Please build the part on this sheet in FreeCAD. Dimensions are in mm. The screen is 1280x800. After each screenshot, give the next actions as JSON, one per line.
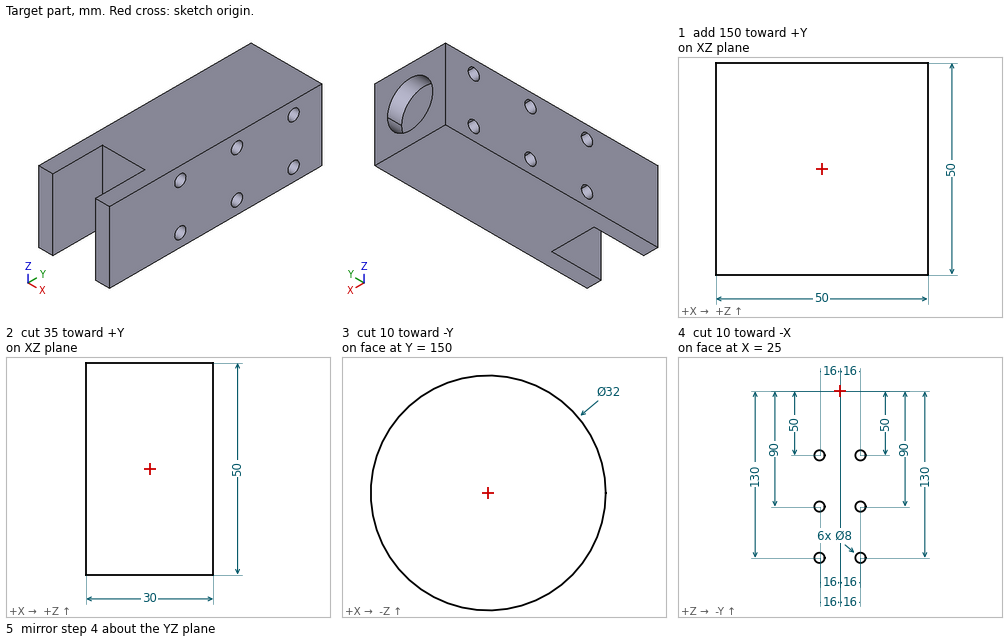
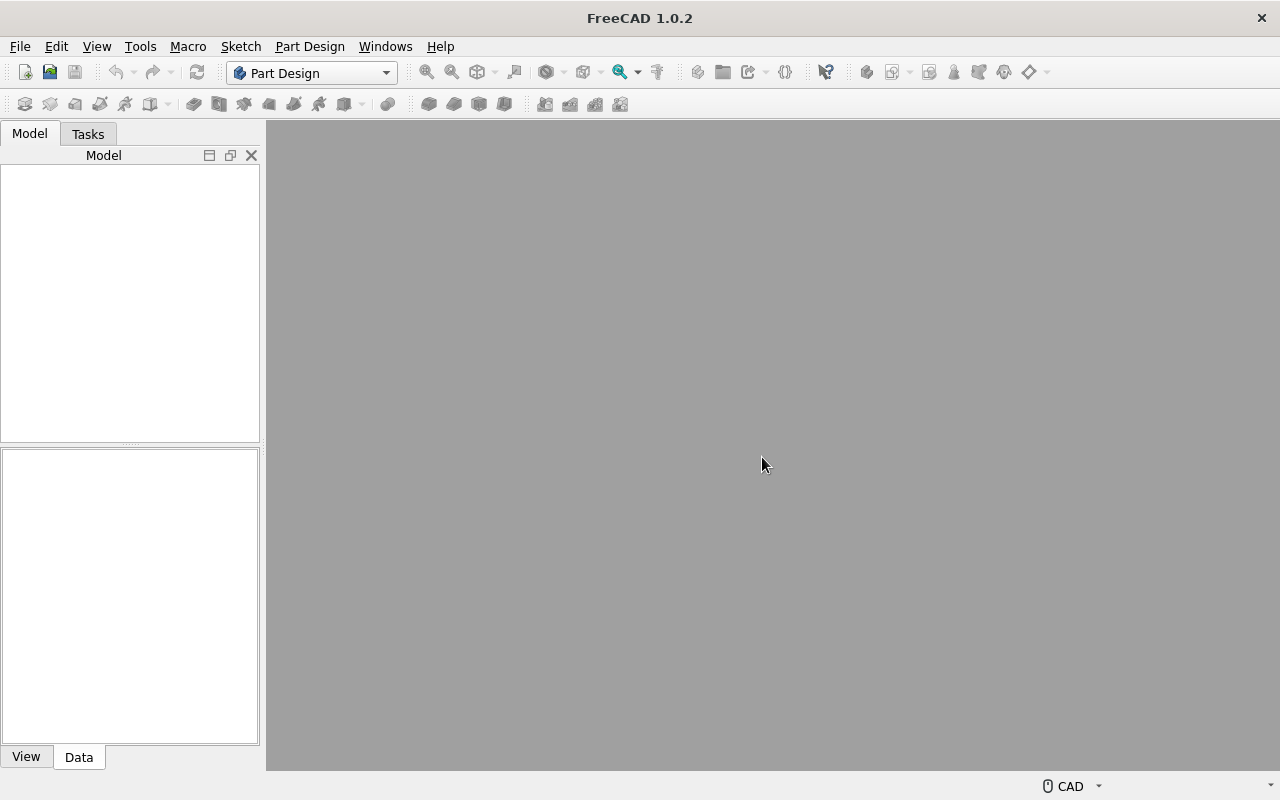
{"action": "left_click", "coordinate": [25, 72]}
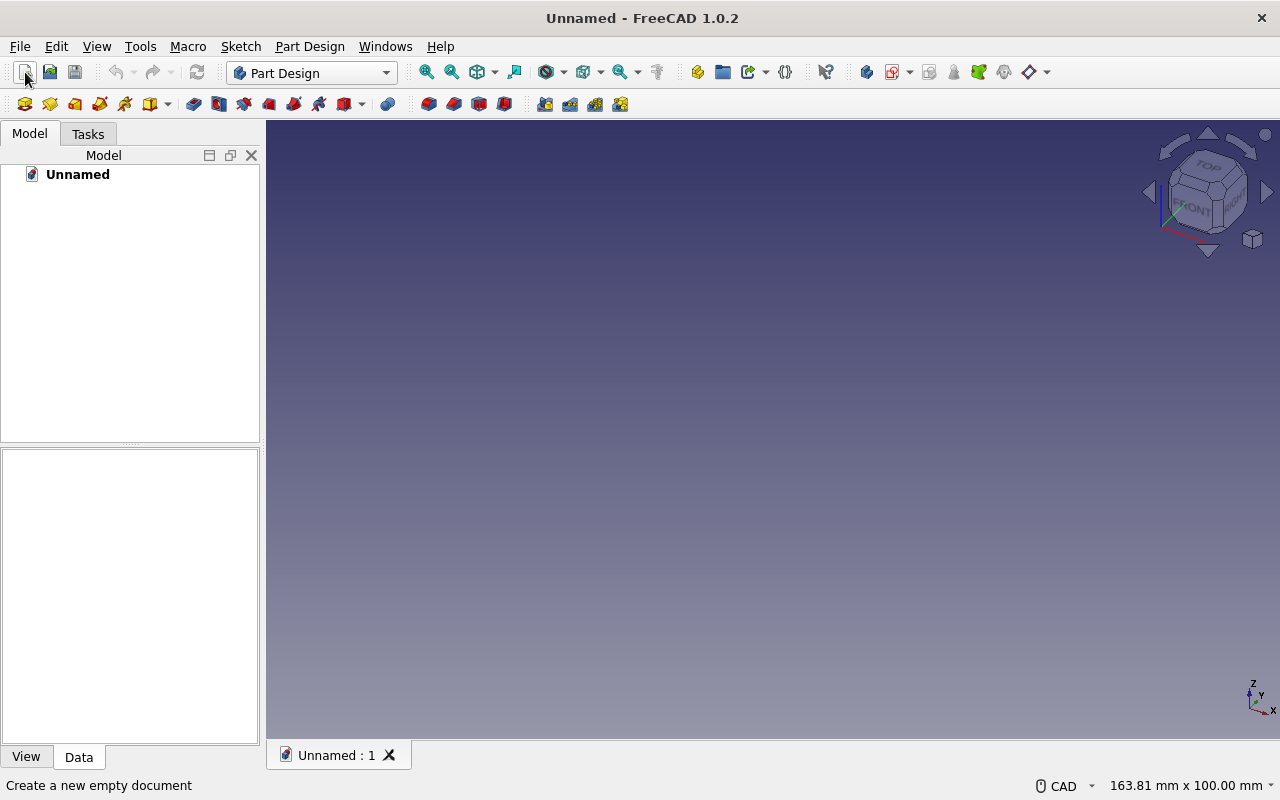
{"action": "left_click", "coordinate": [892, 72]}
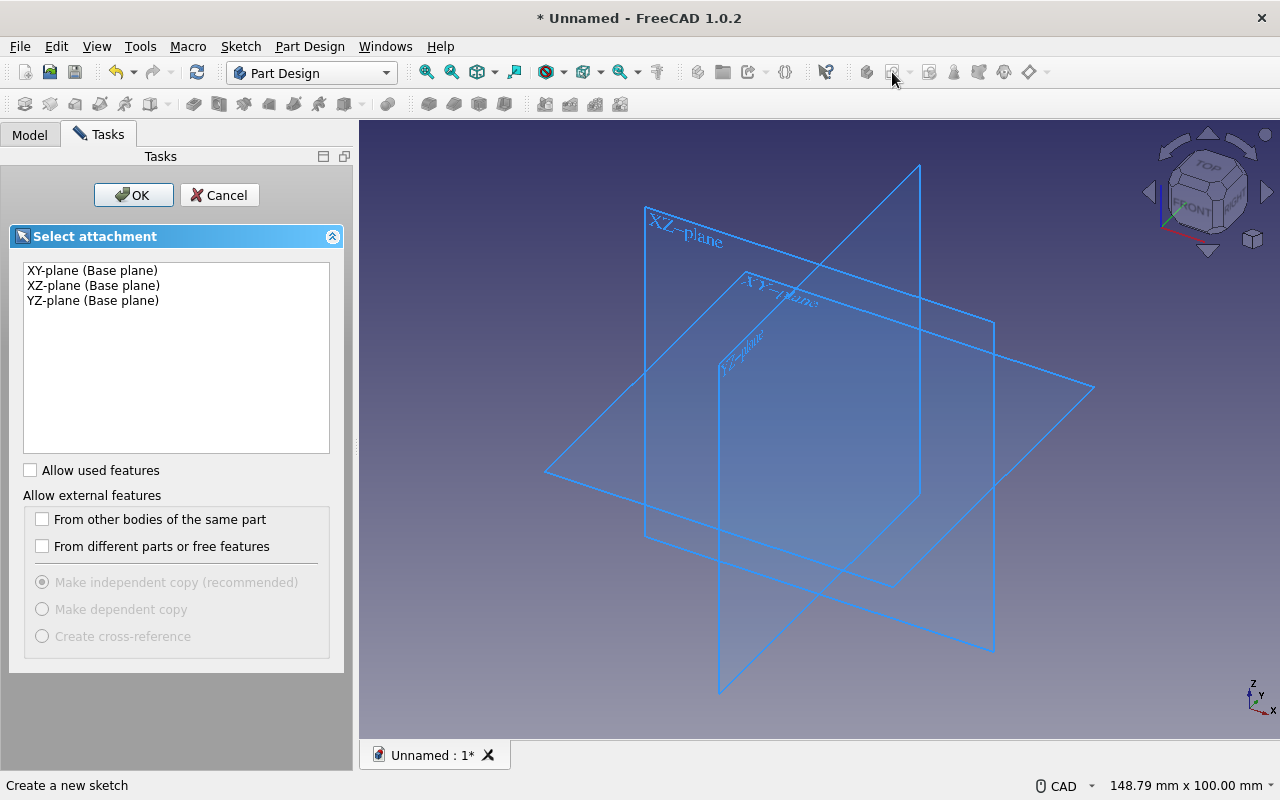
{"action": "left_click", "coordinate": [84, 286]}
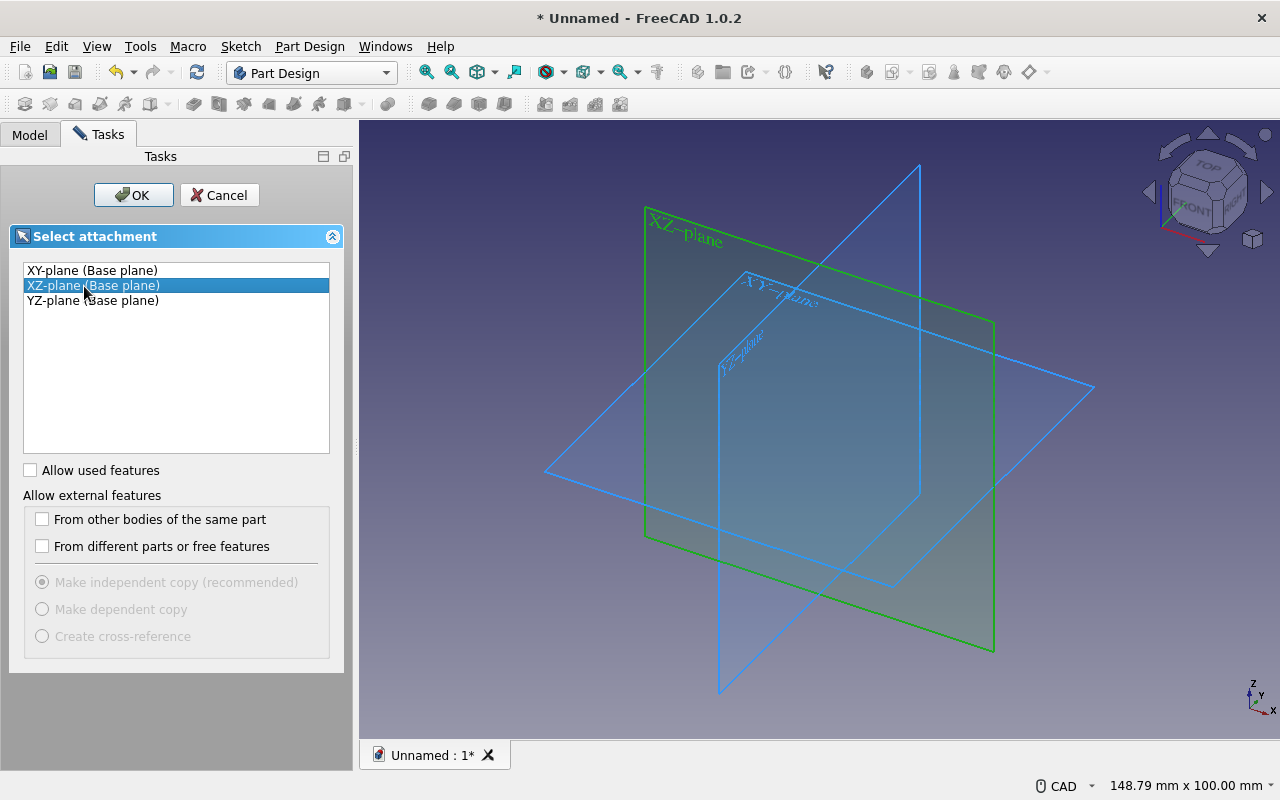
{"action": "left_click", "coordinate": [134, 195]}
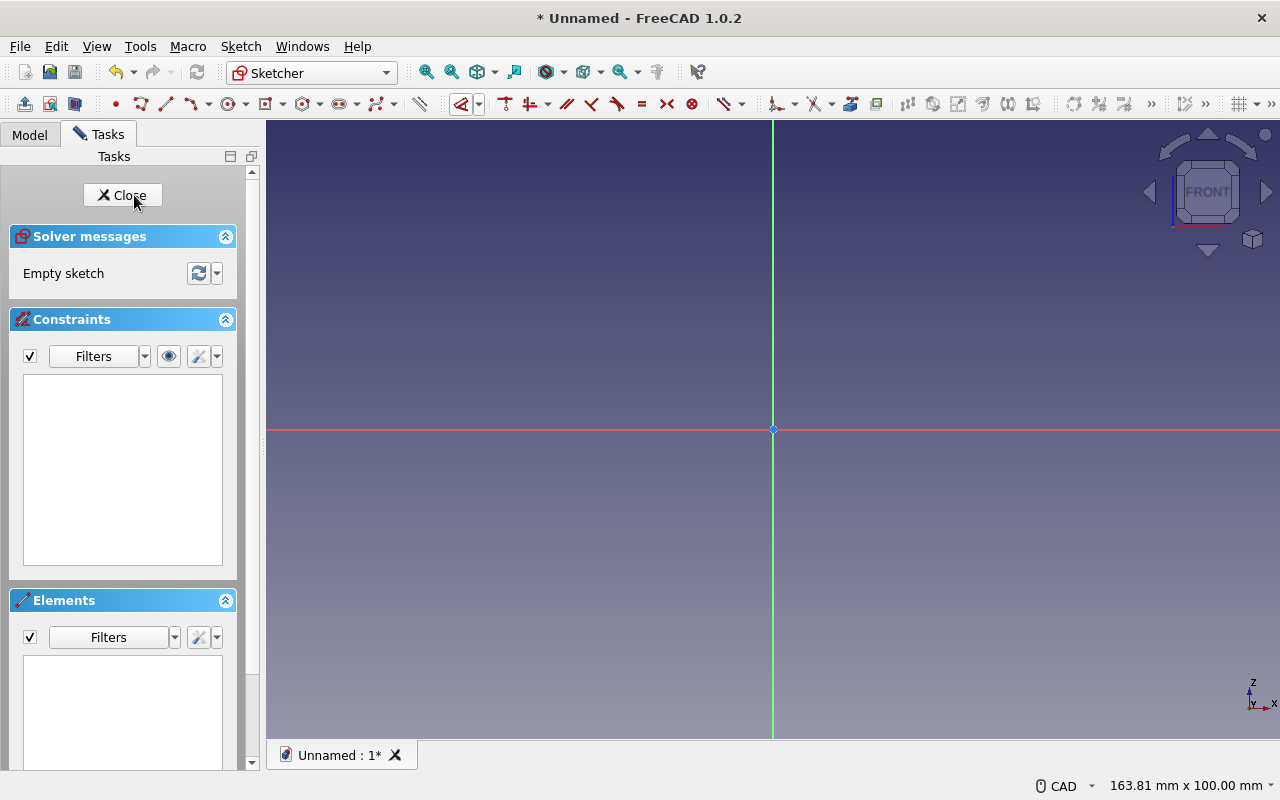
{"action": "left_click", "coordinate": [264, 104]}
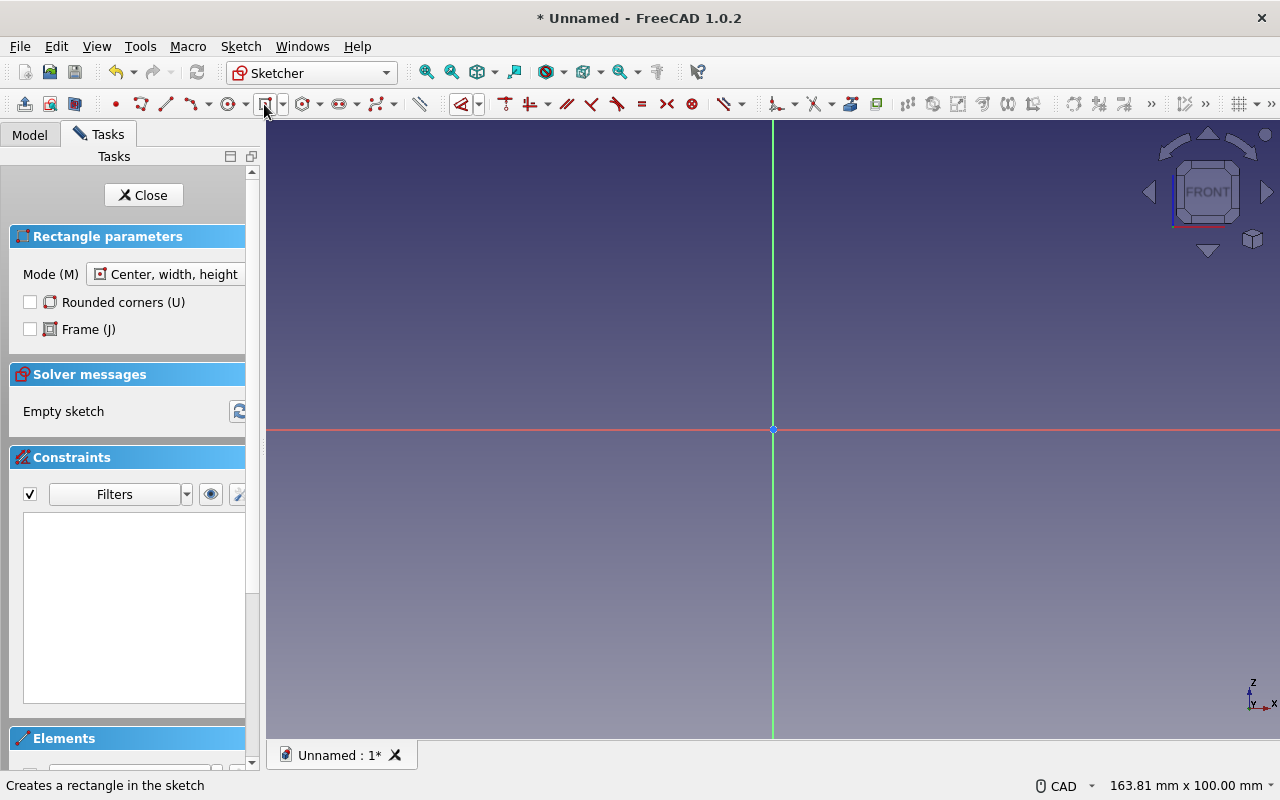
{"action": "left_click", "coordinate": [773, 430]}
{"action": "mouse_move", "coordinate": [928, 275]}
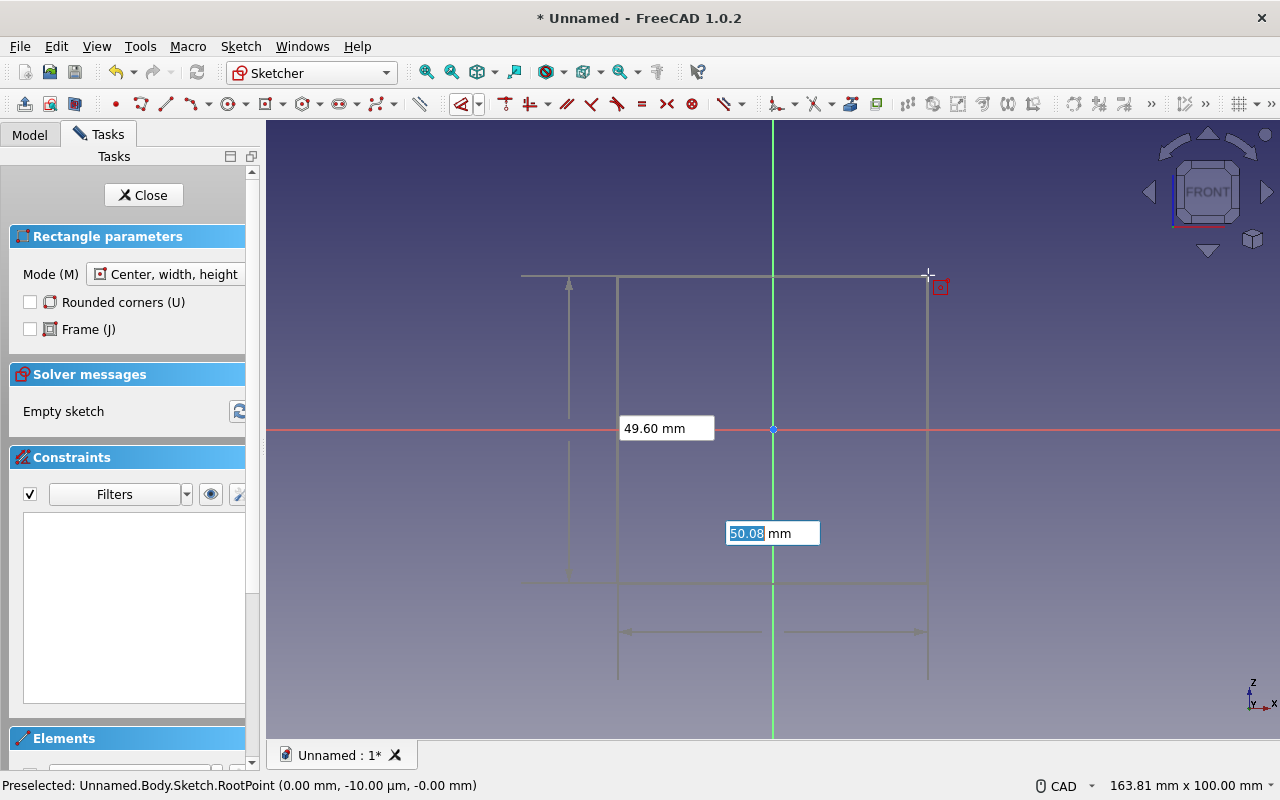
{"action": "type", "text": "50"}
{"action": "key", "text": "Tab"}
{"action": "type", "text": "50"}
{"action": "key", "text": "Return"}
{"action": "key", "text": "Escape"}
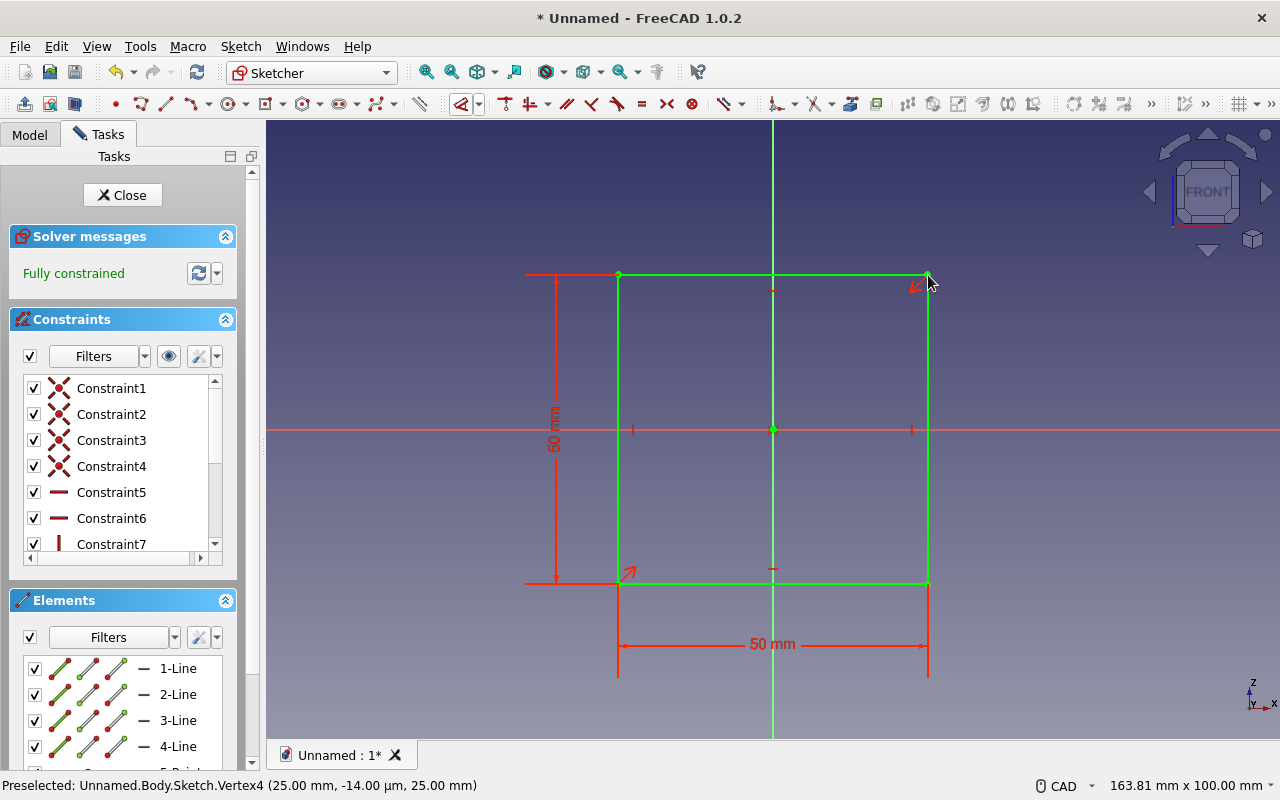
{"action": "left_click", "coordinate": [123, 195]}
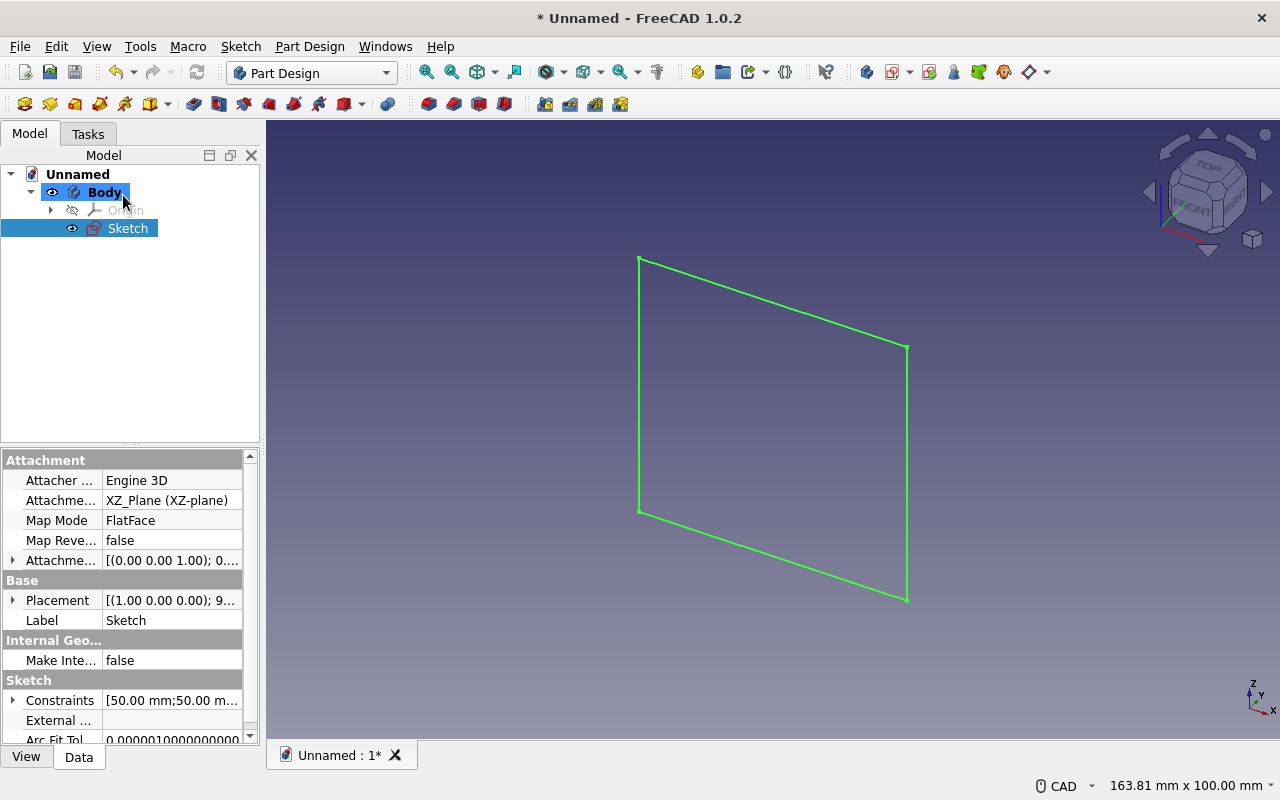
{"action": "left_click", "coordinate": [25, 104]}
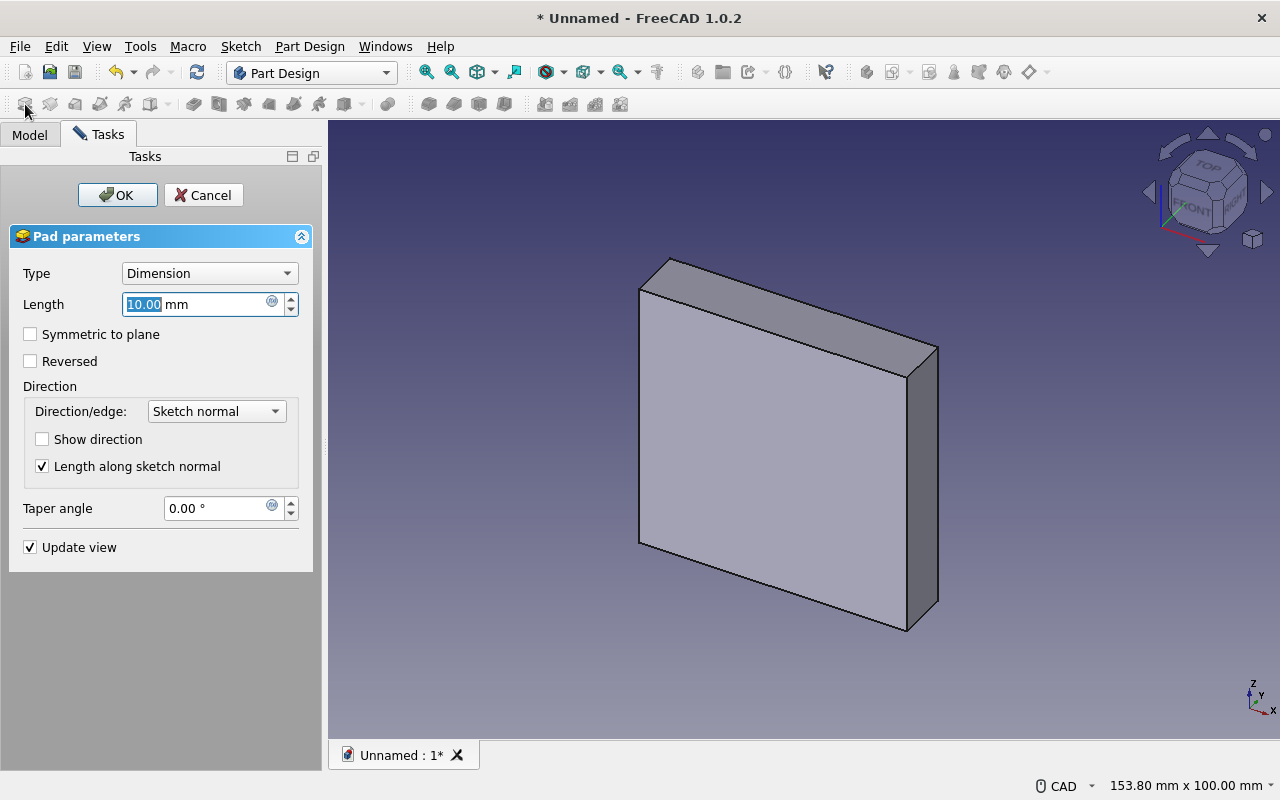
{"action": "type", "text": "150"}
{"action": "key", "text": "Tab"}